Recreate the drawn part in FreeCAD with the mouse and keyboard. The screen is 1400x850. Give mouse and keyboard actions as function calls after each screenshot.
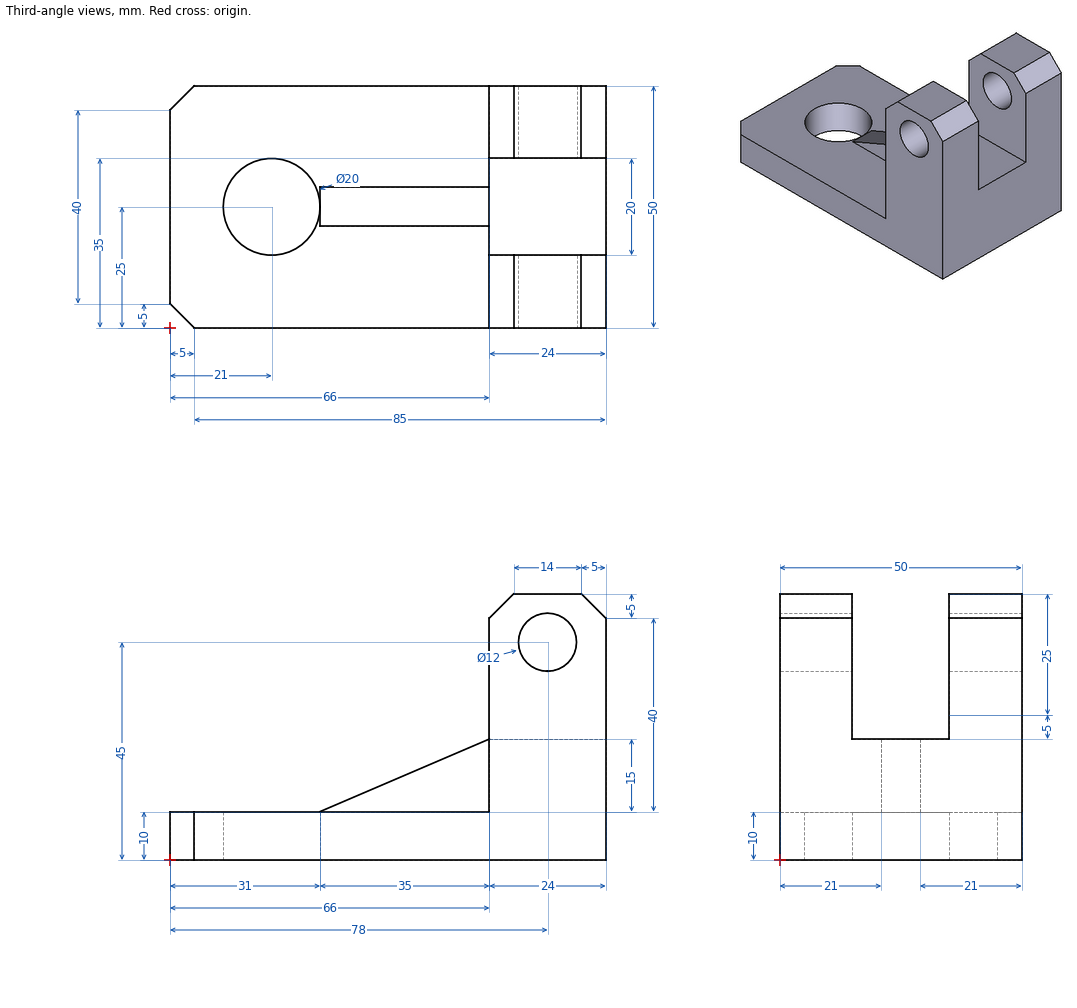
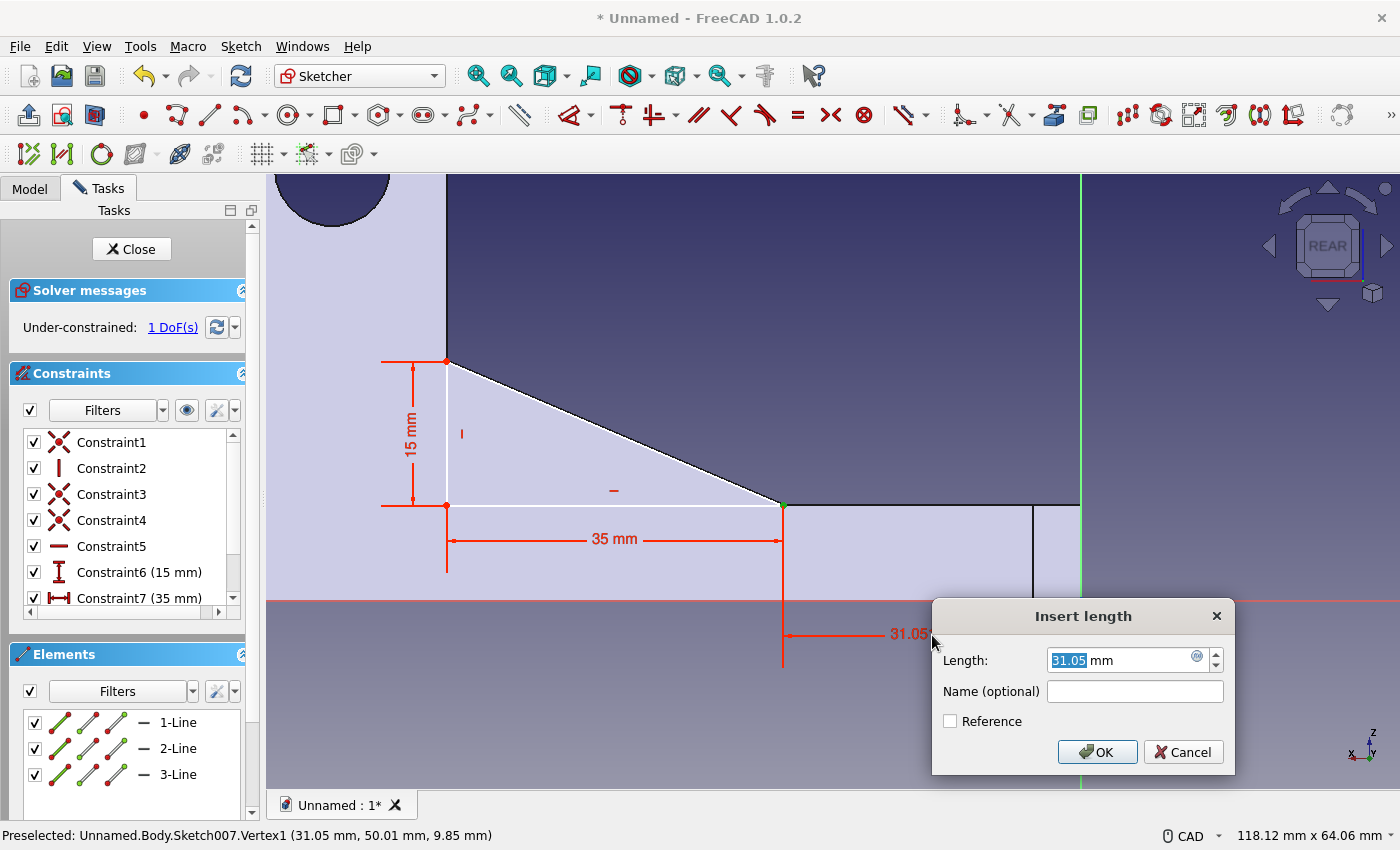
text(31)
key(Return)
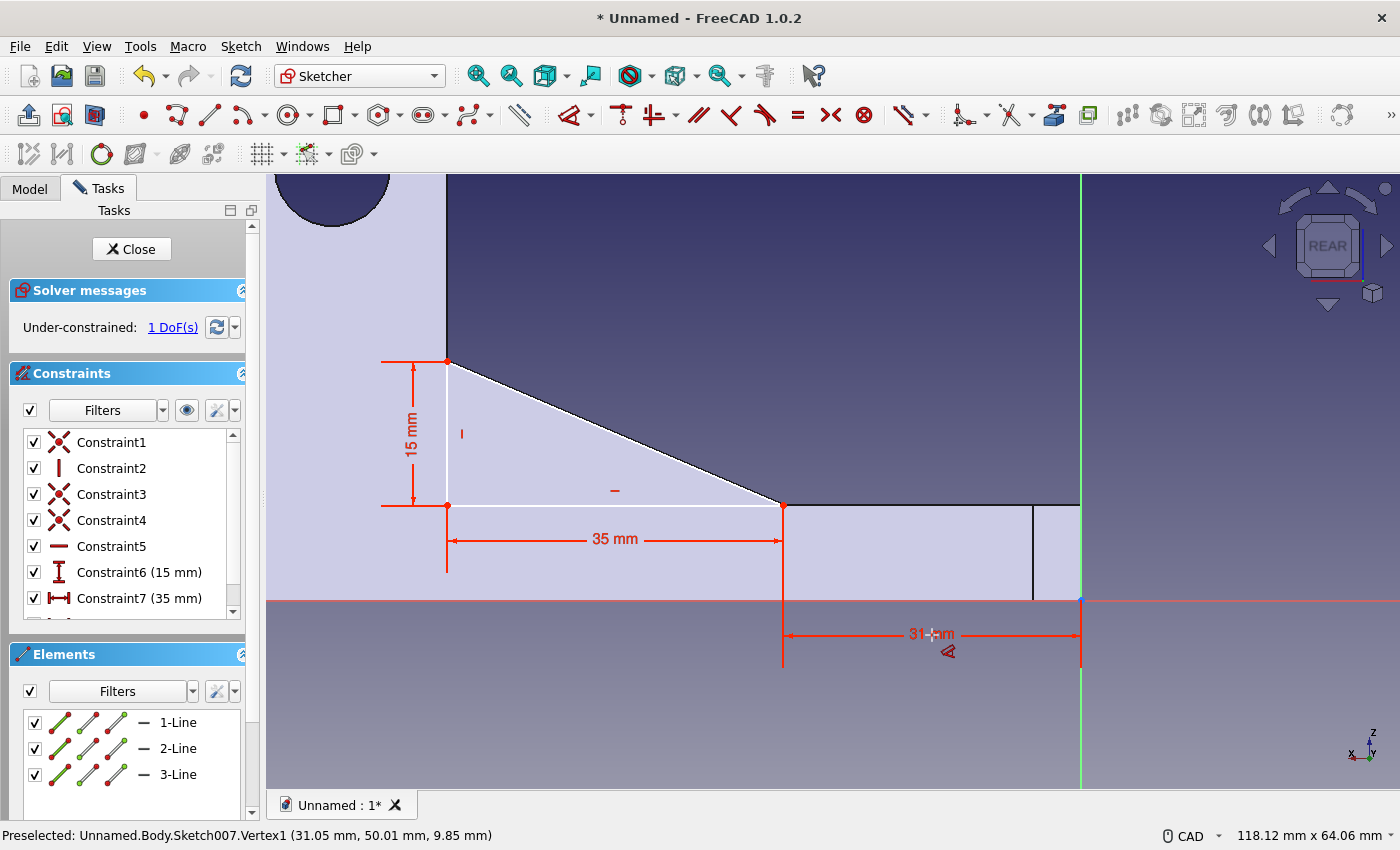
click(783, 506)
click(1115, 553)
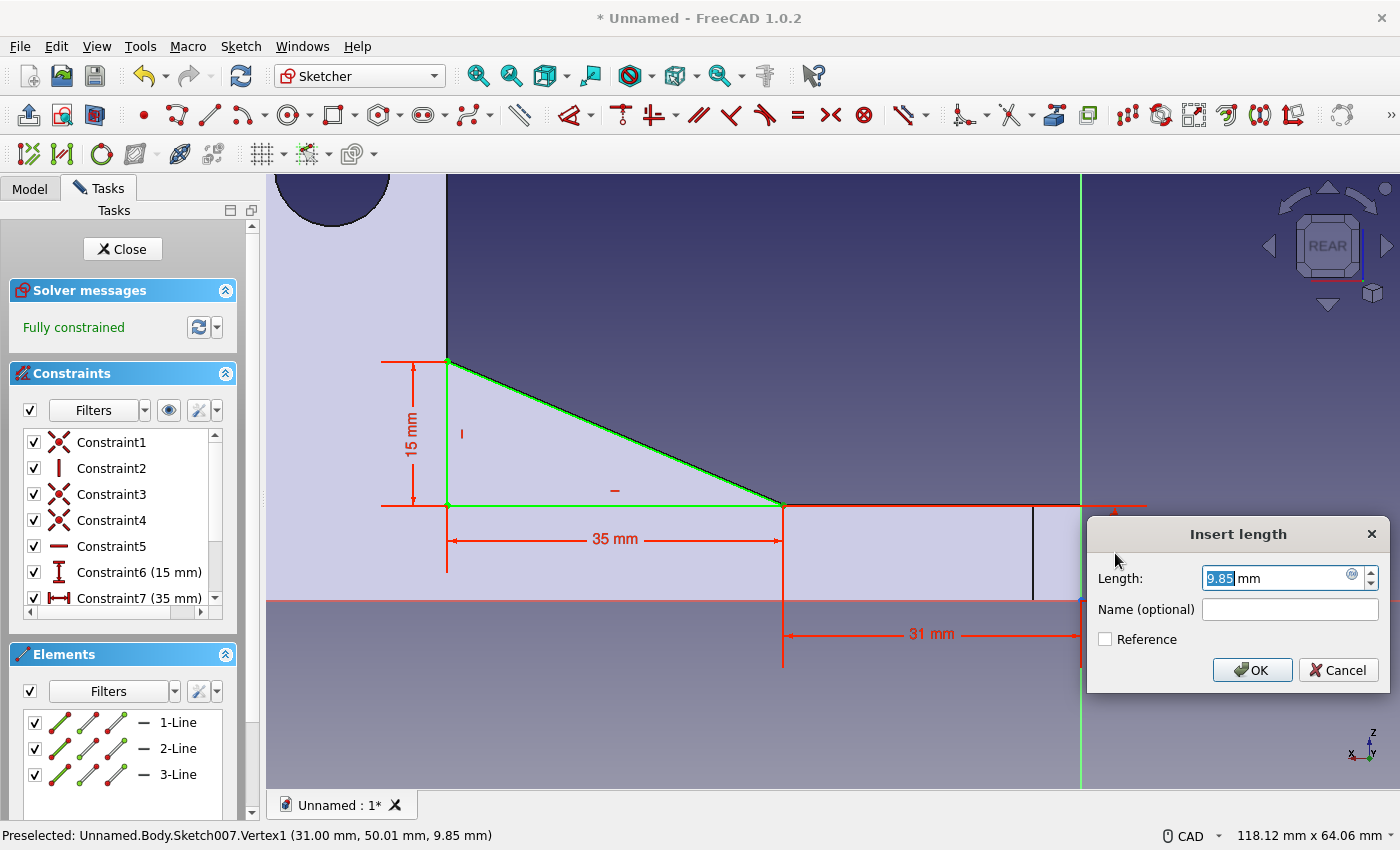
text(10)
key(Return)
key(Escape)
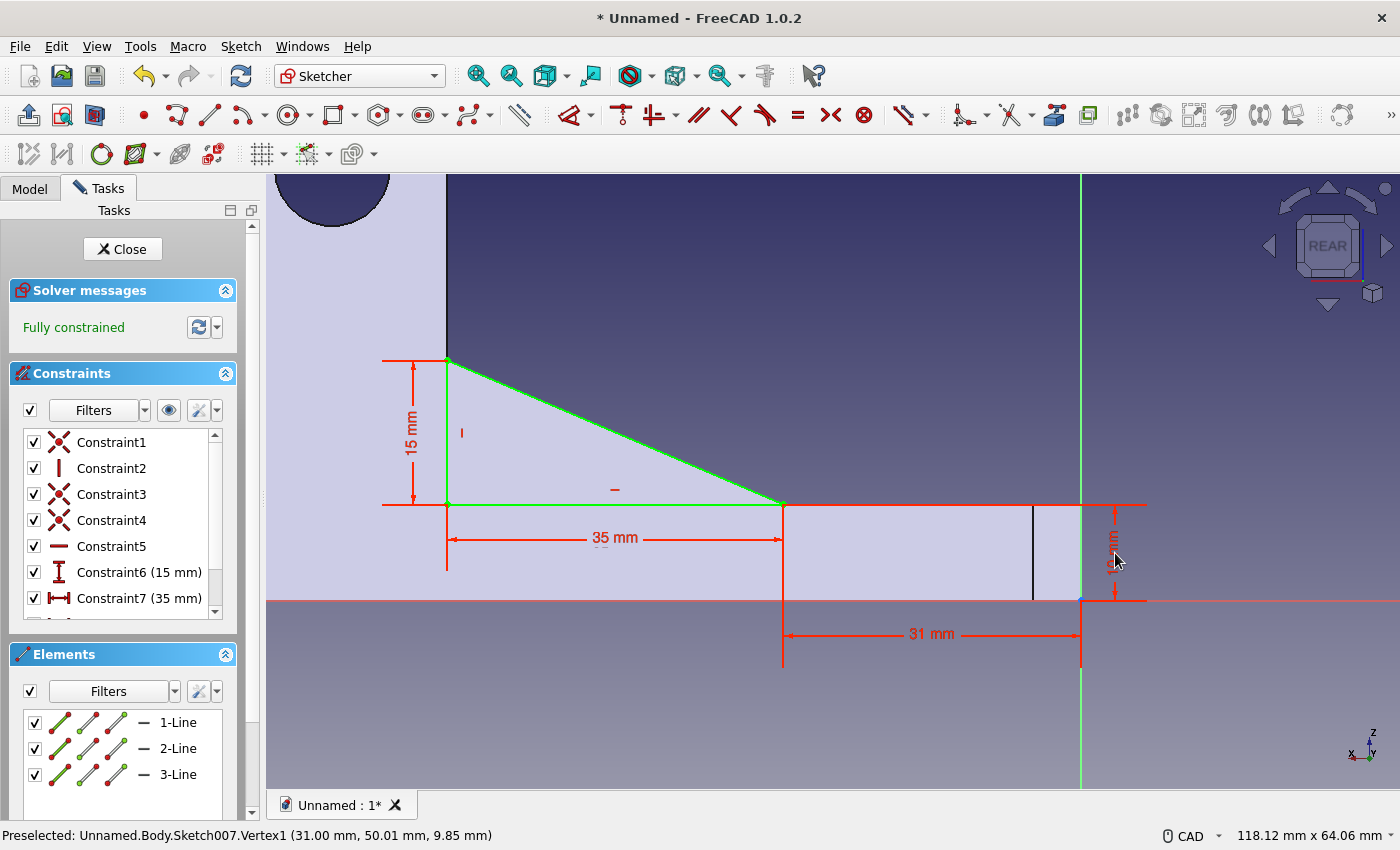
click(123, 249)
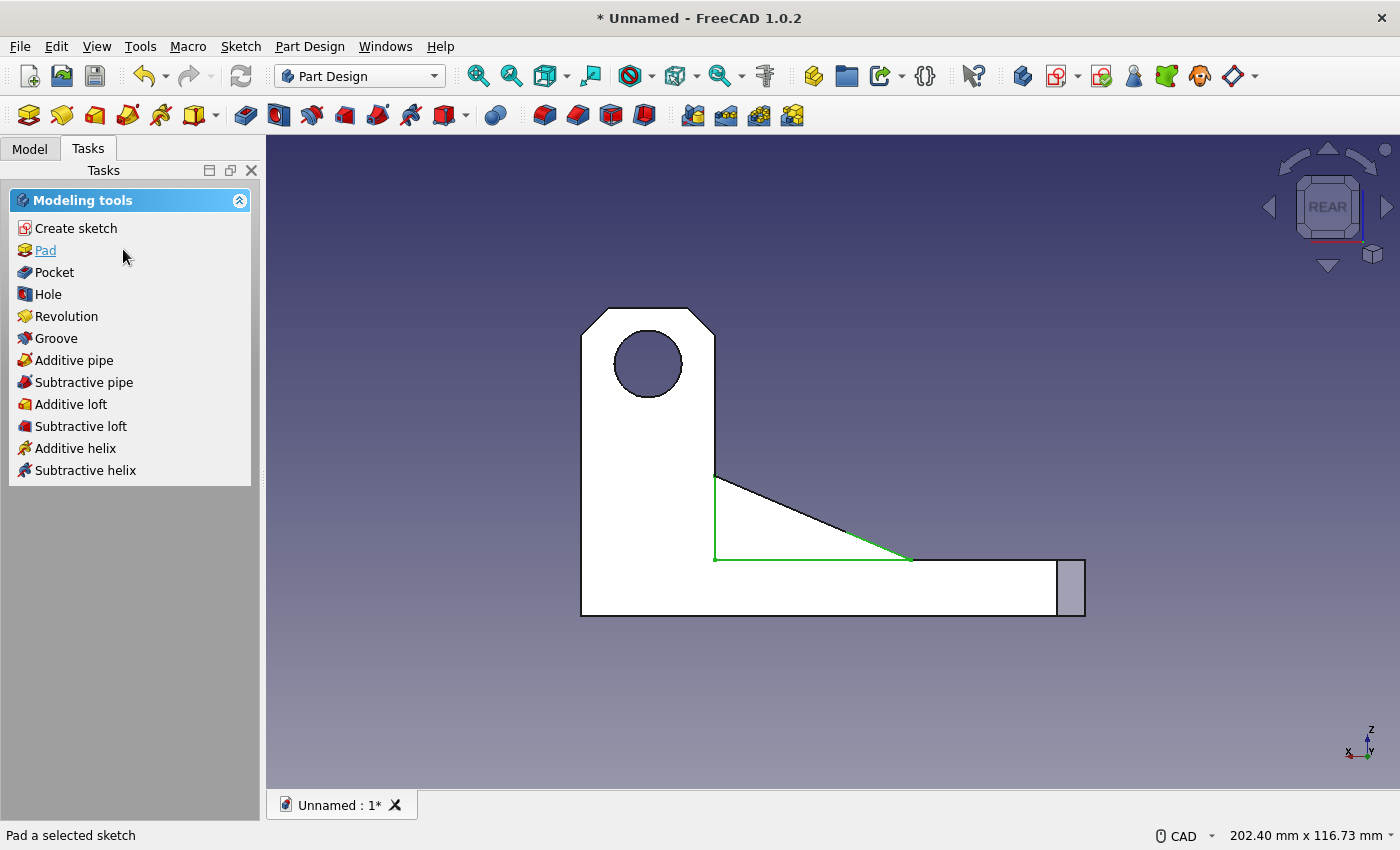
click(246, 116)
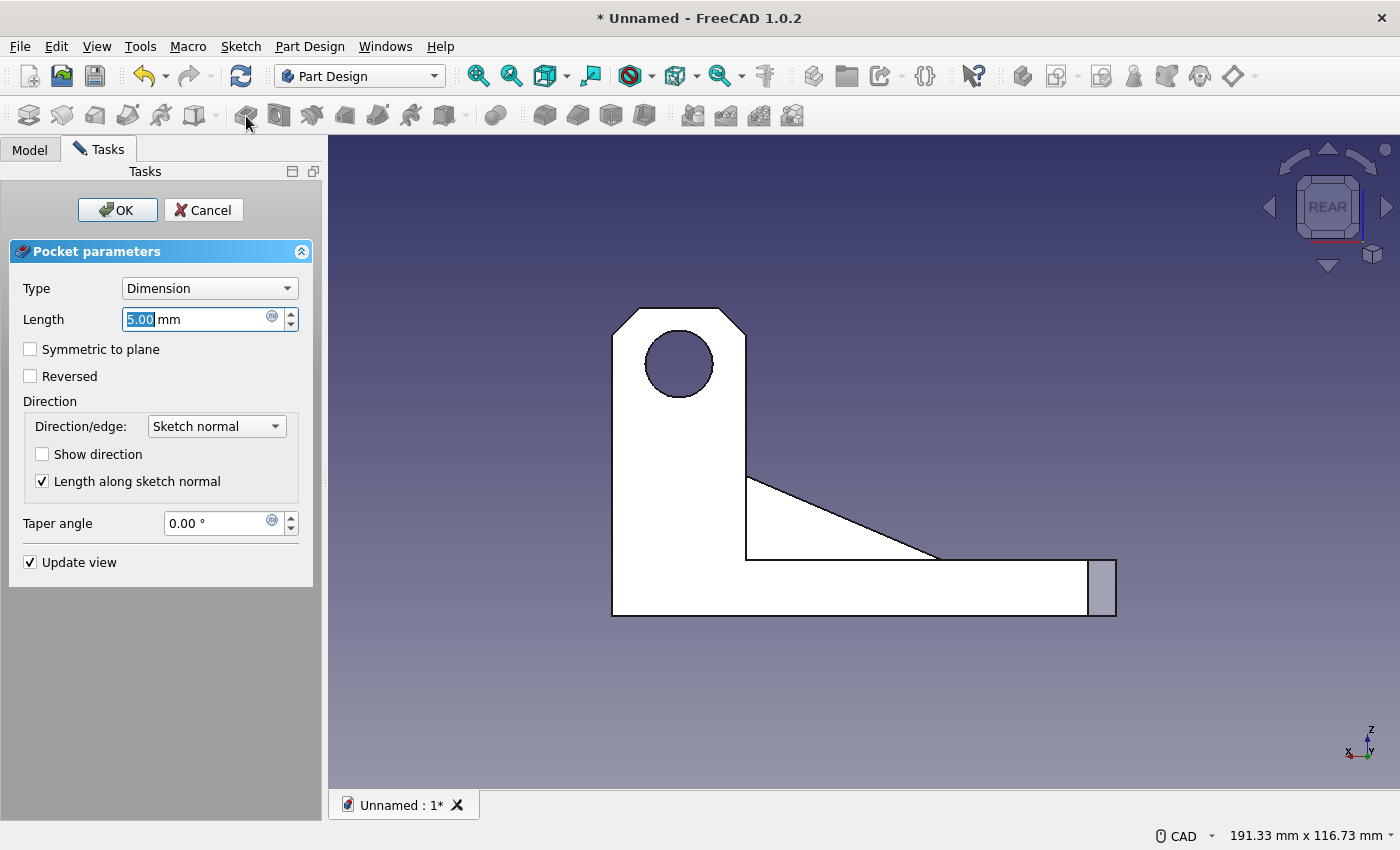
text(21)
key(Tab)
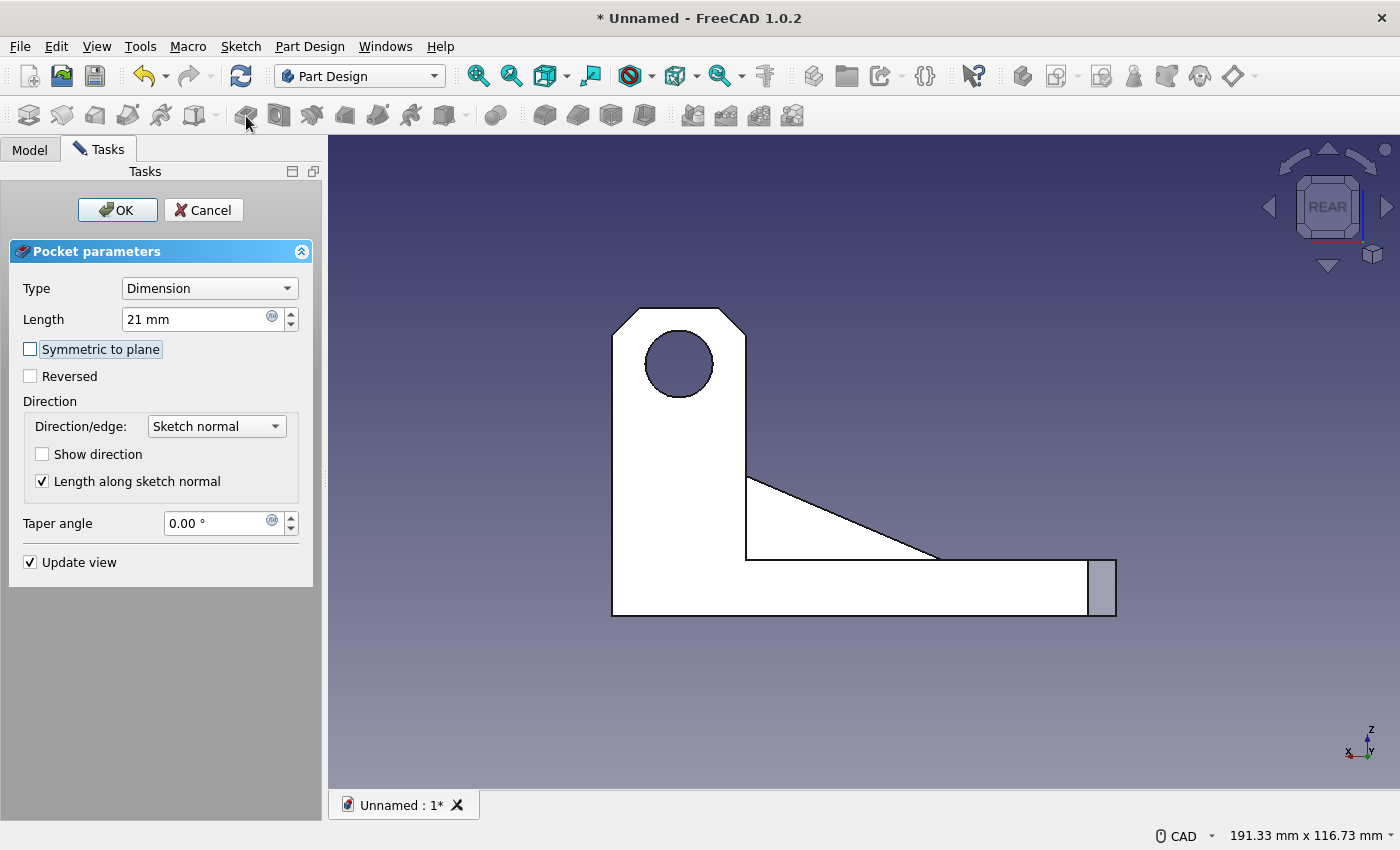
click(118, 210)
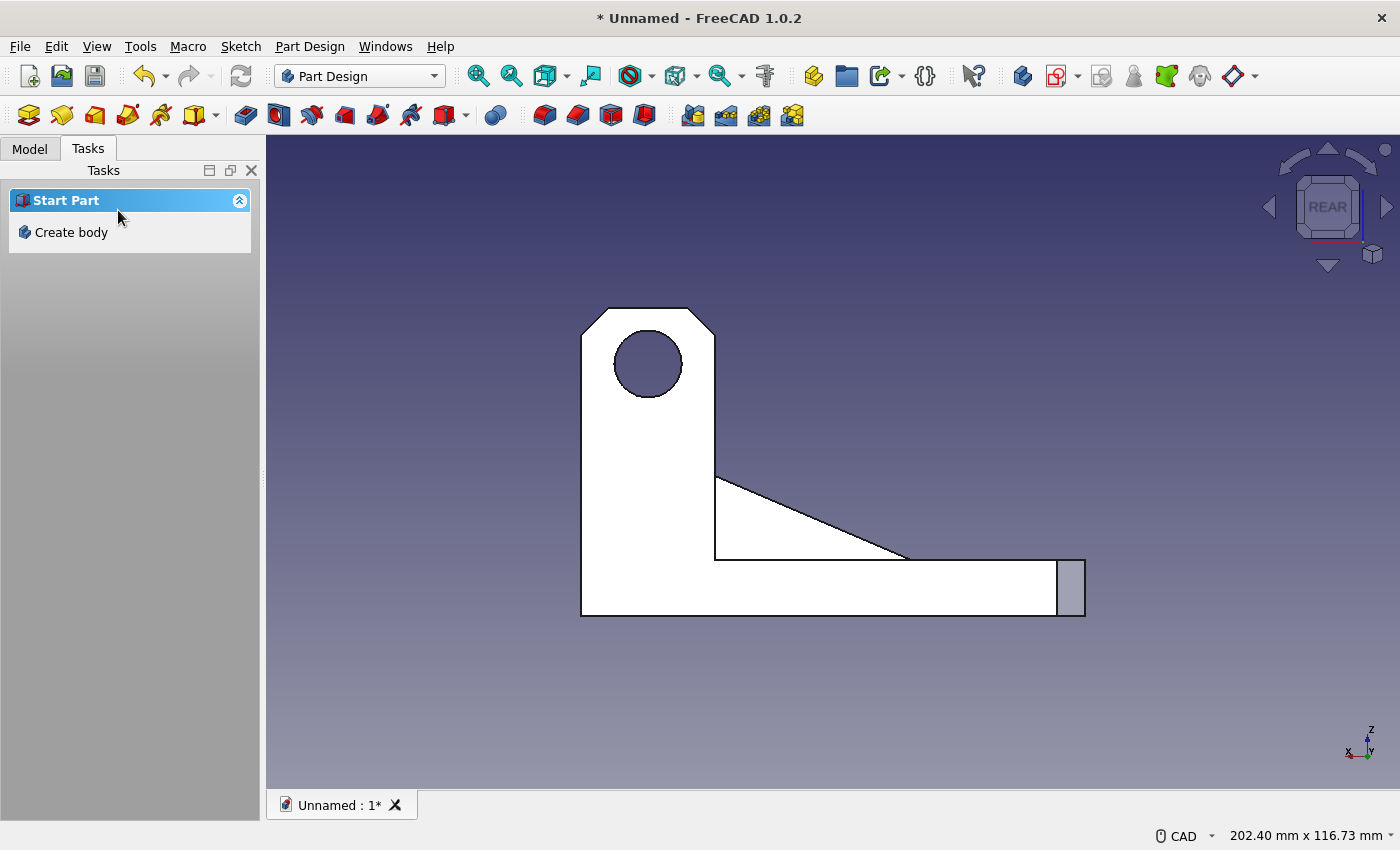
key(0)